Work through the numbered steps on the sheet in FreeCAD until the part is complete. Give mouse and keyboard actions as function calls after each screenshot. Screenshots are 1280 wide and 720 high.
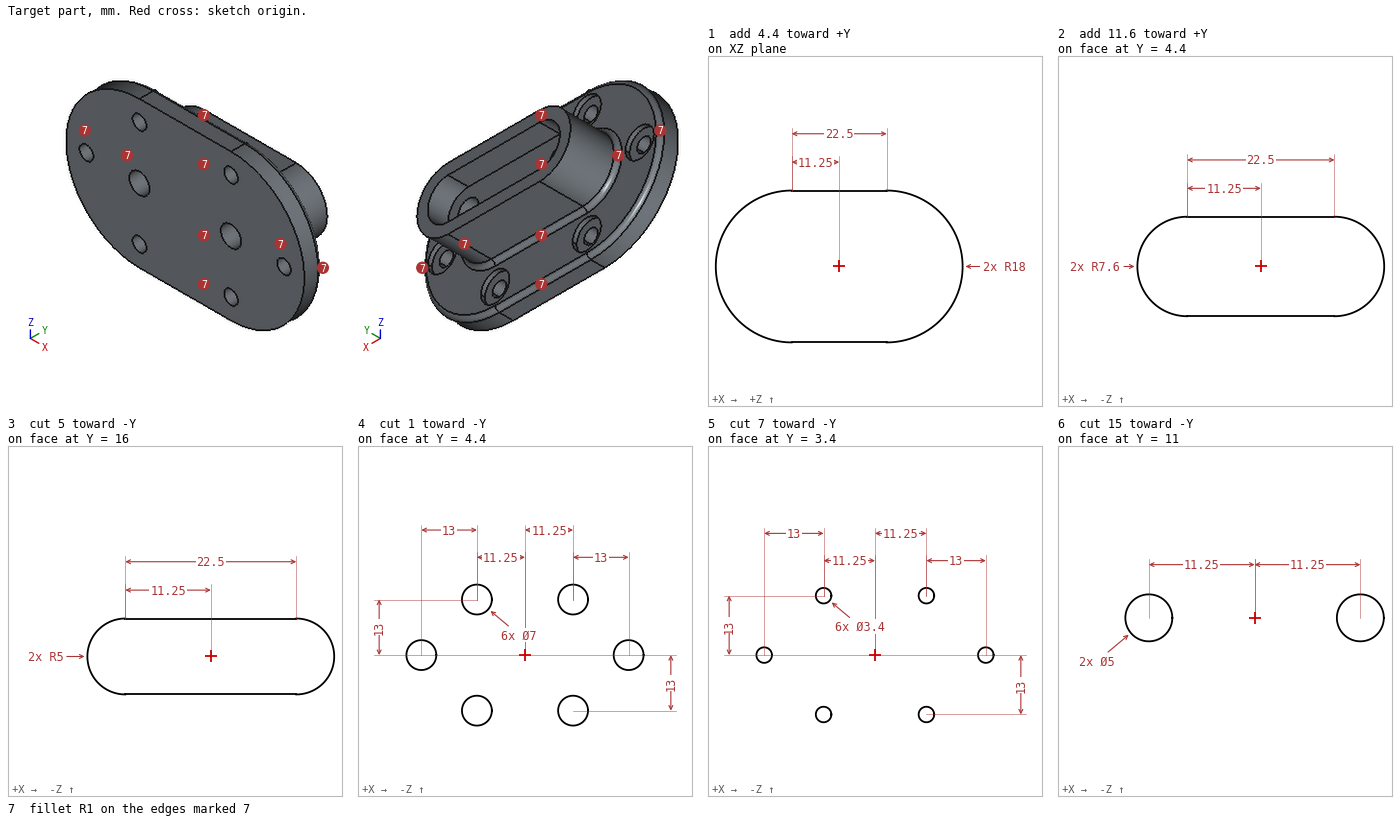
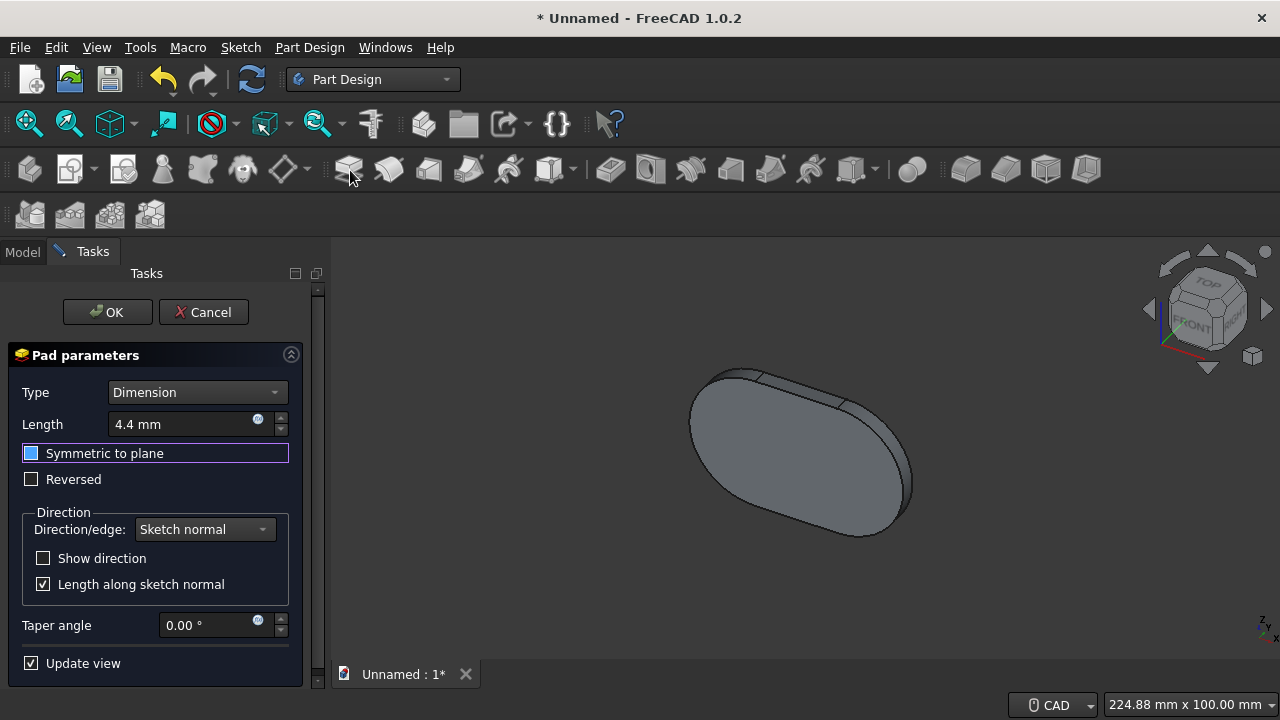
click(30, 479)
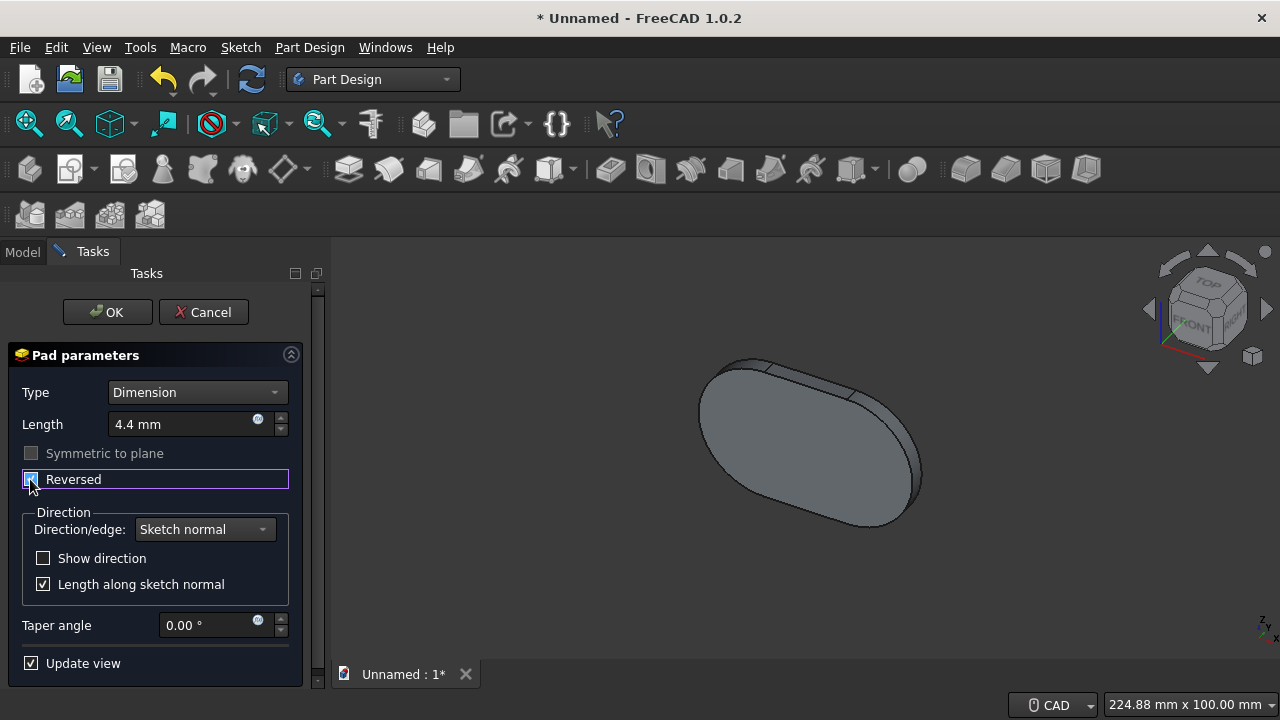
click(108, 312)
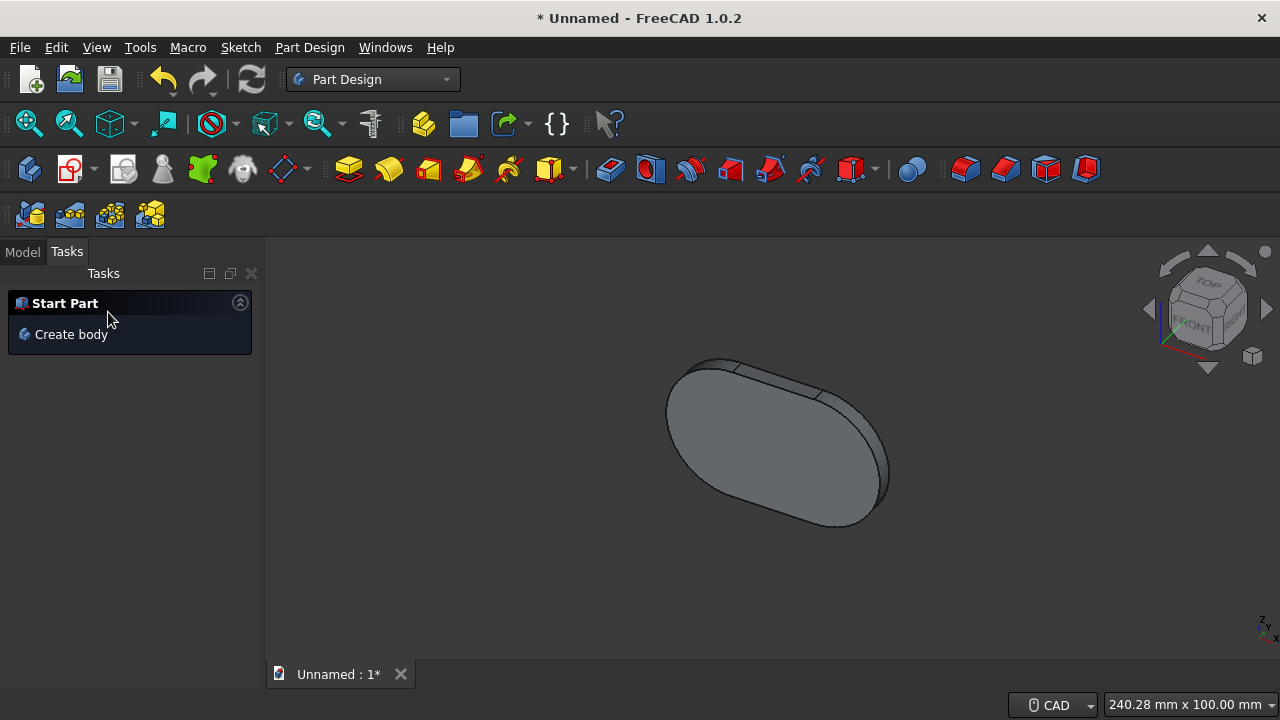
key(4)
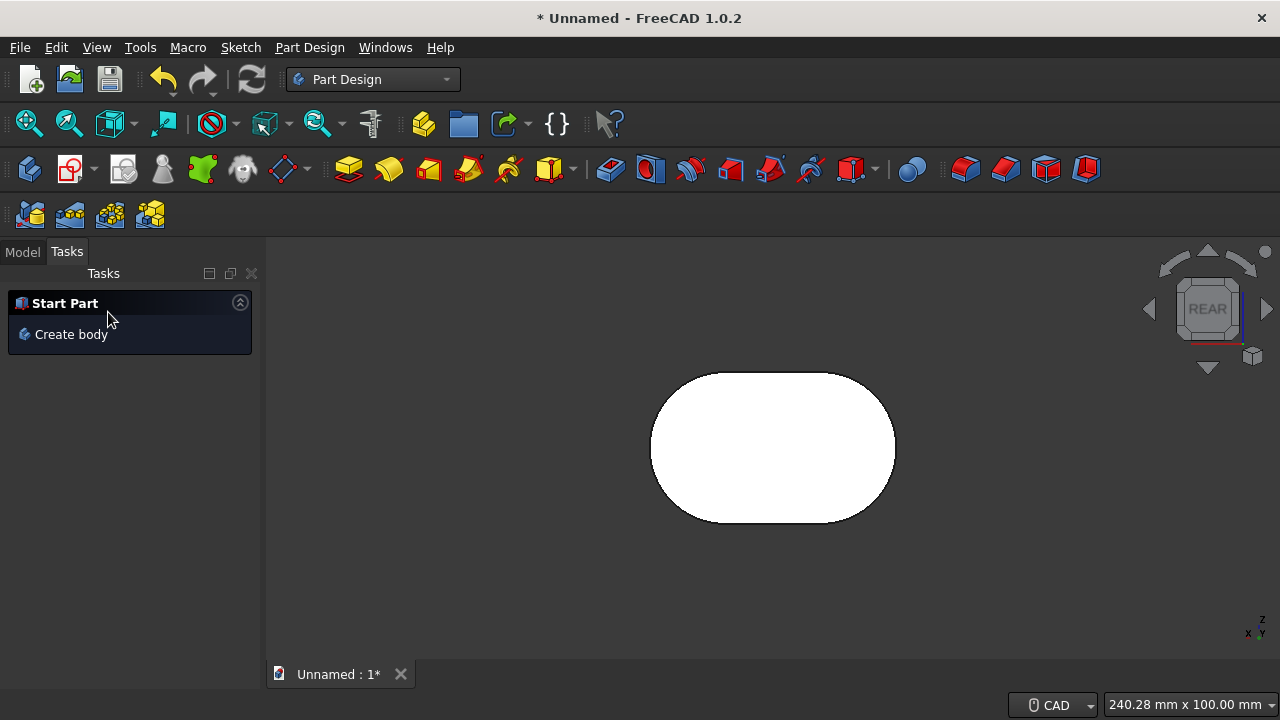
click(30, 124)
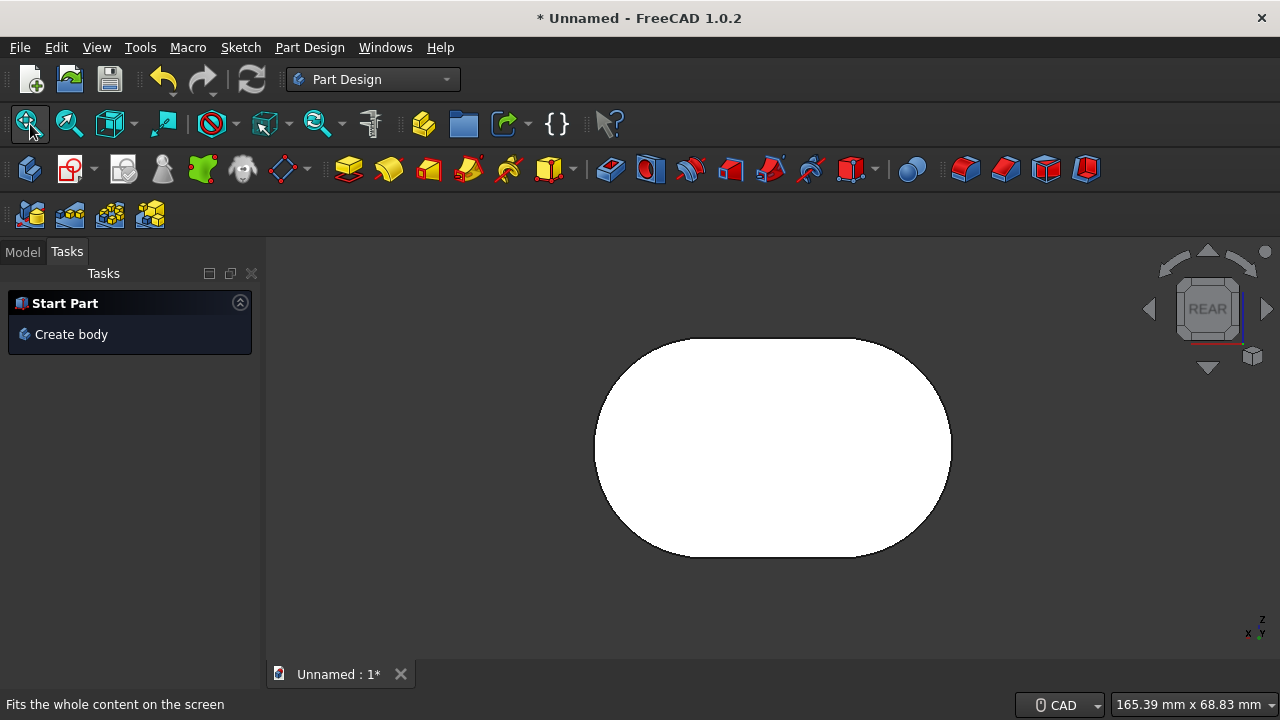
click(824, 447)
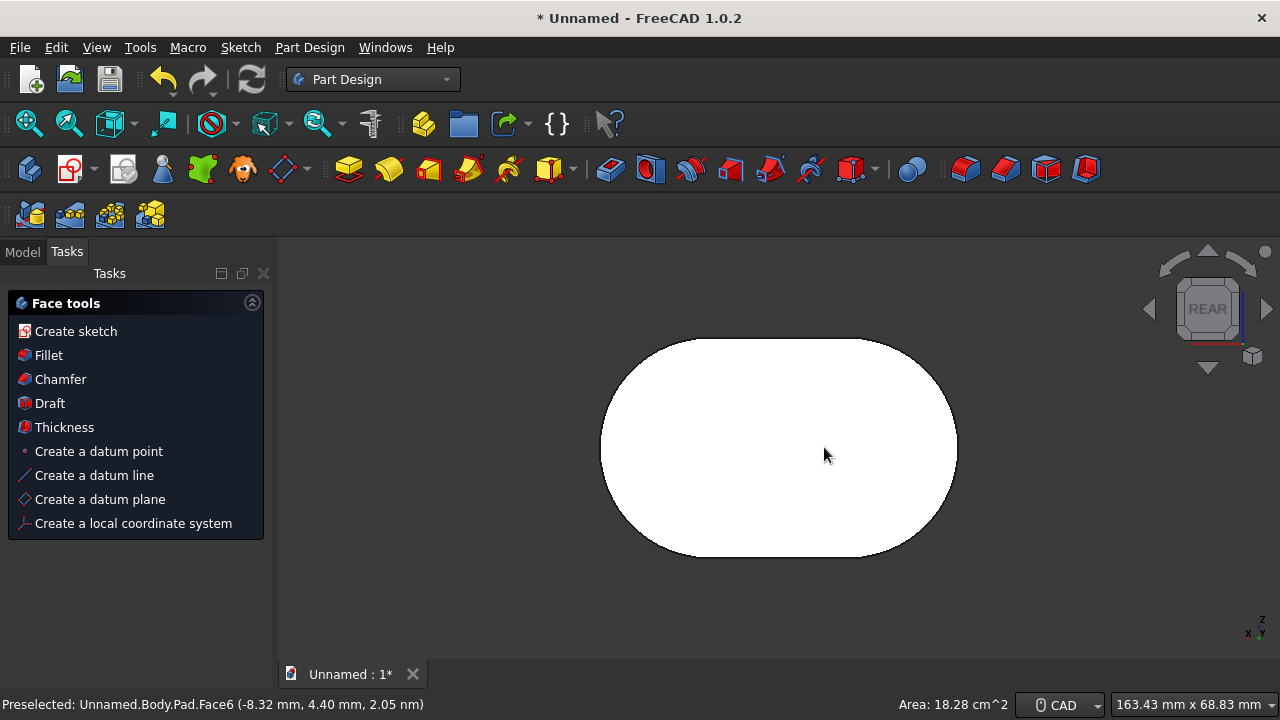
click(70, 170)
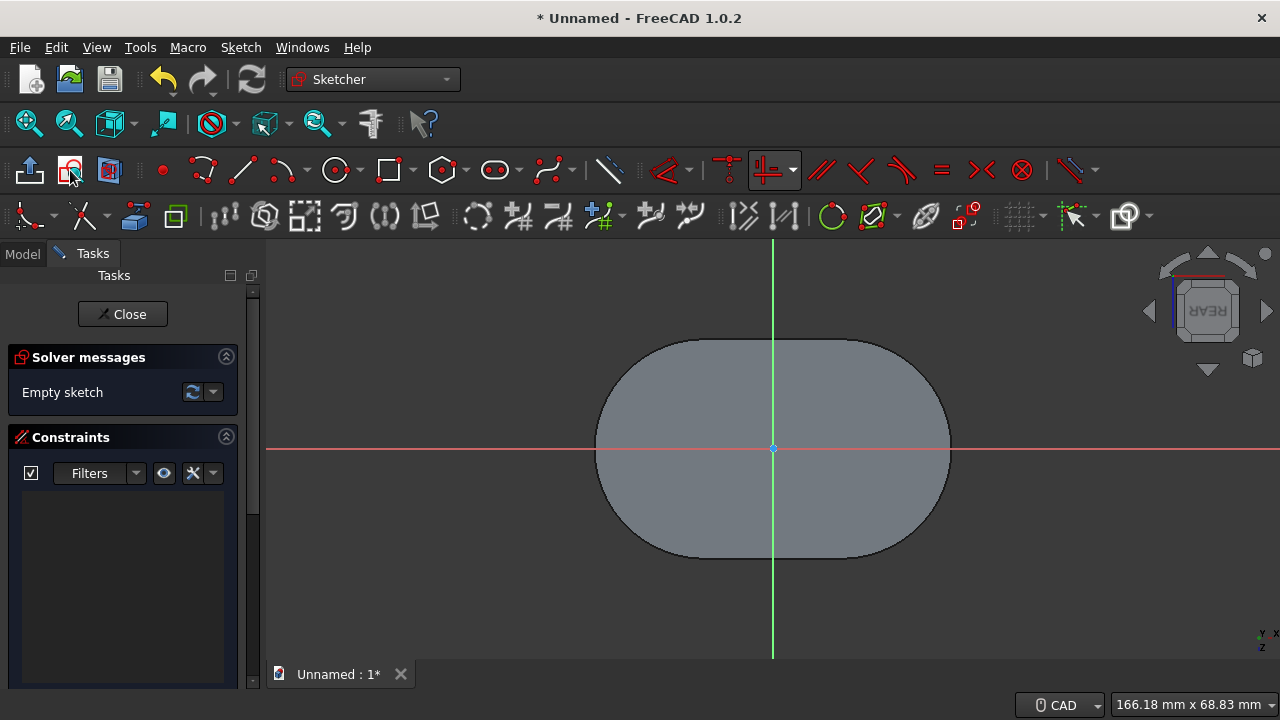
scroll(813, 449, up, 5)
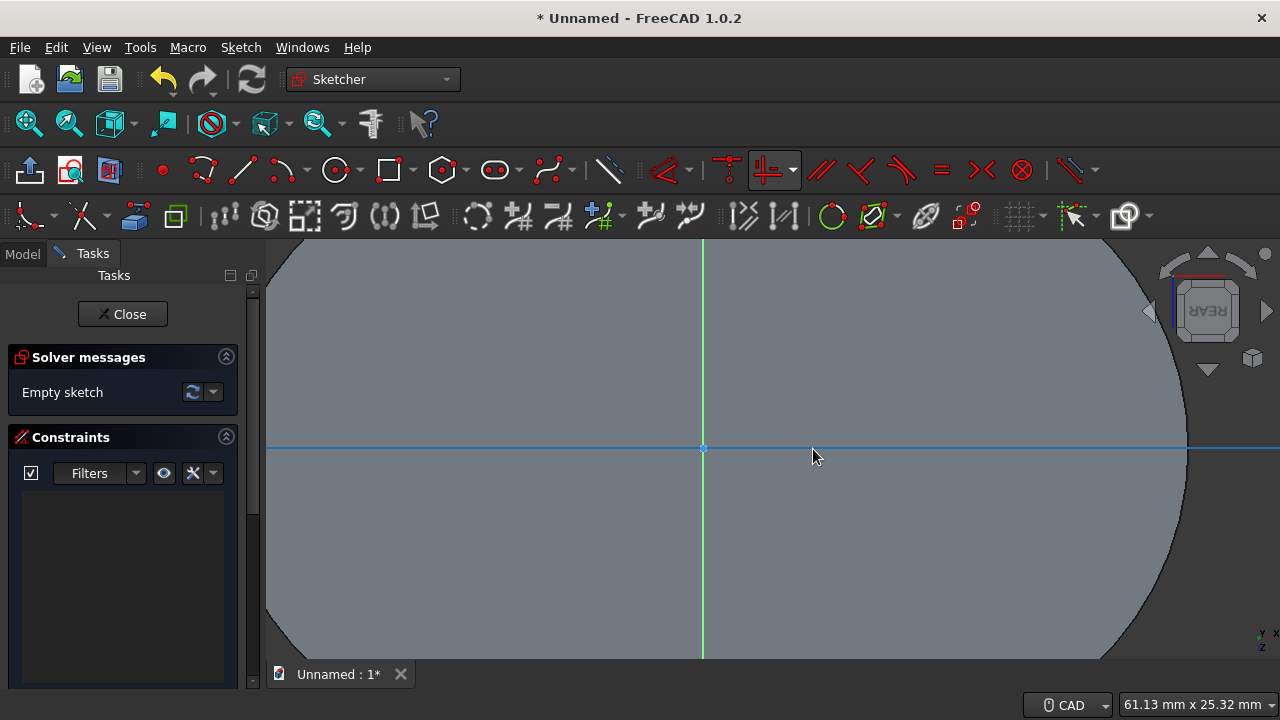
click(496, 170)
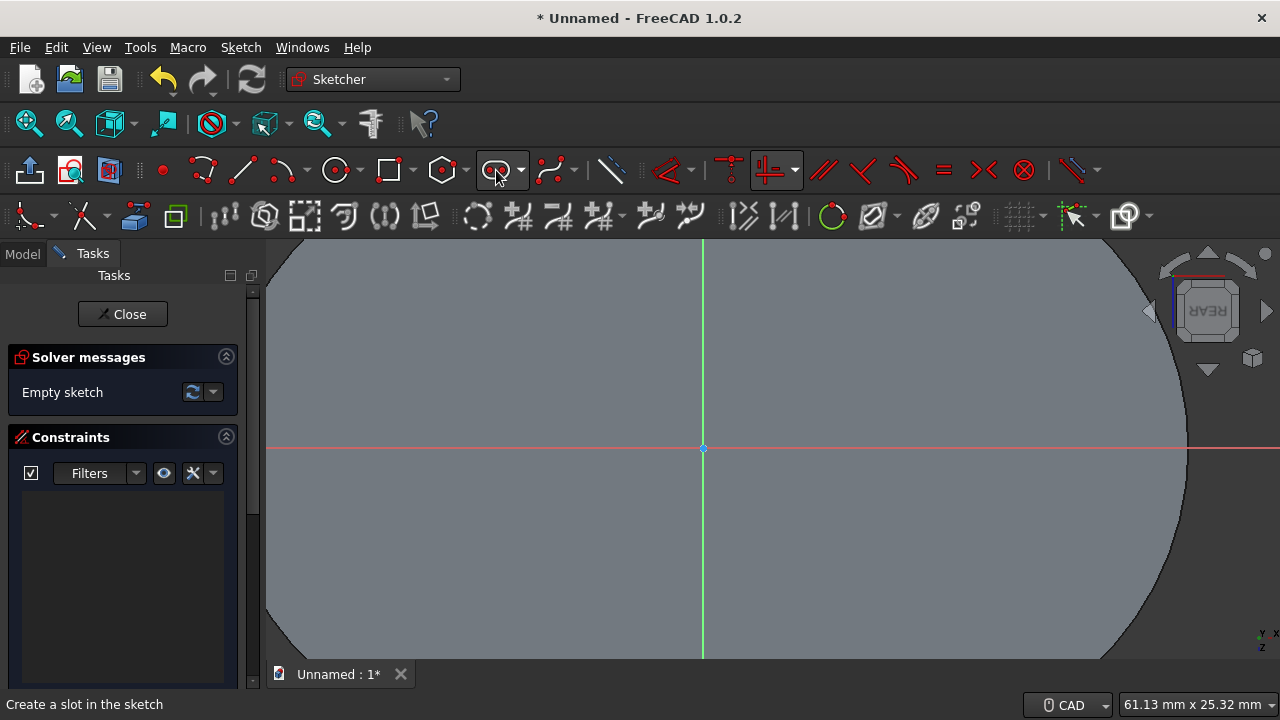
click(517, 448)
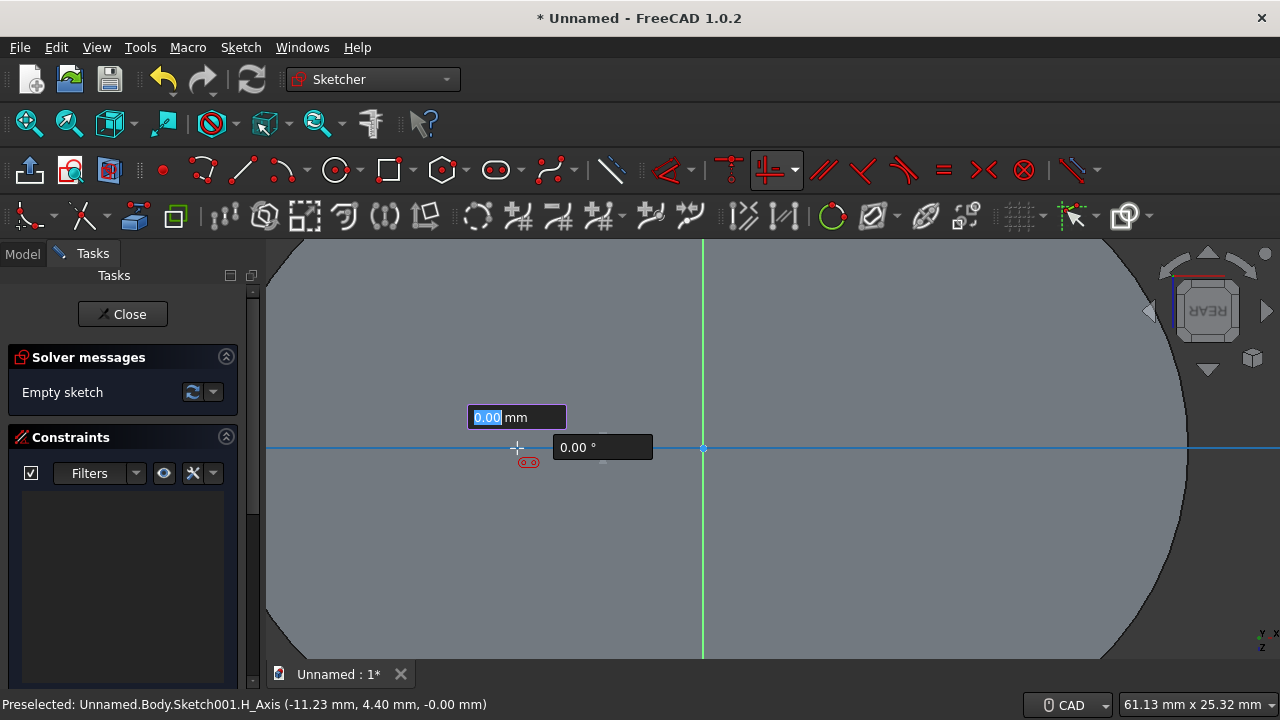
click(890, 439)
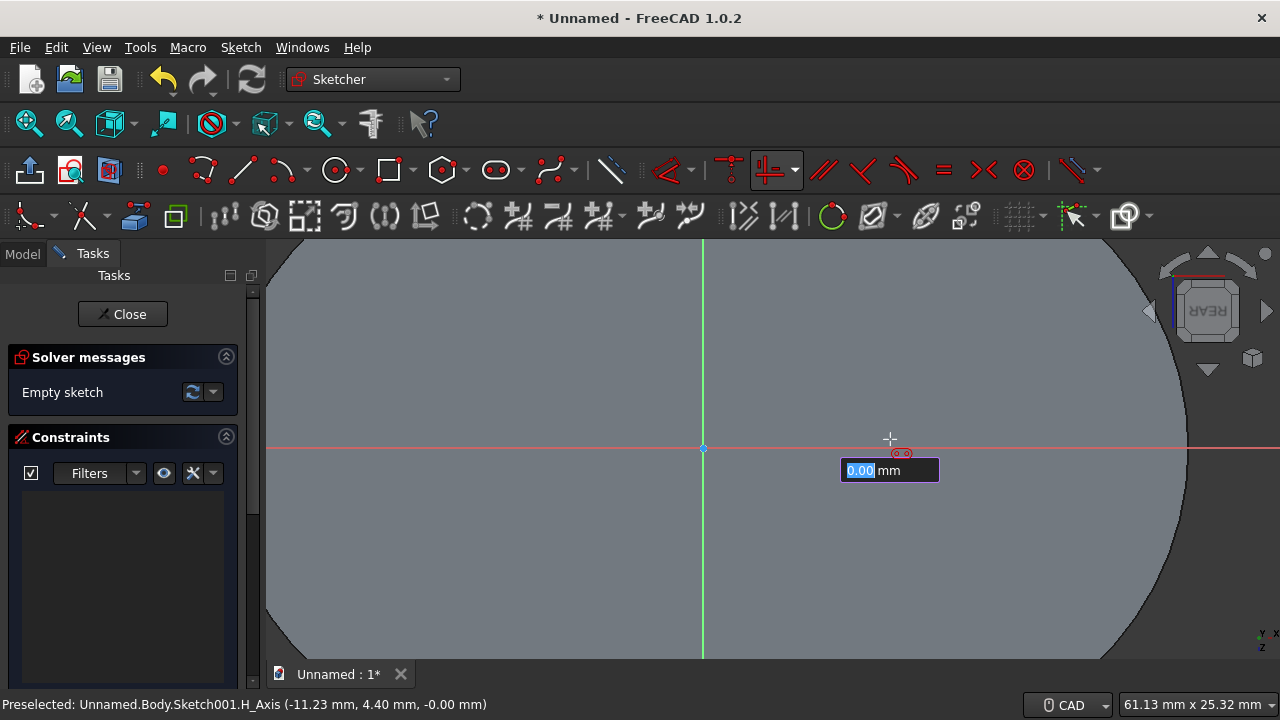
click(759, 322)
key(Escape)